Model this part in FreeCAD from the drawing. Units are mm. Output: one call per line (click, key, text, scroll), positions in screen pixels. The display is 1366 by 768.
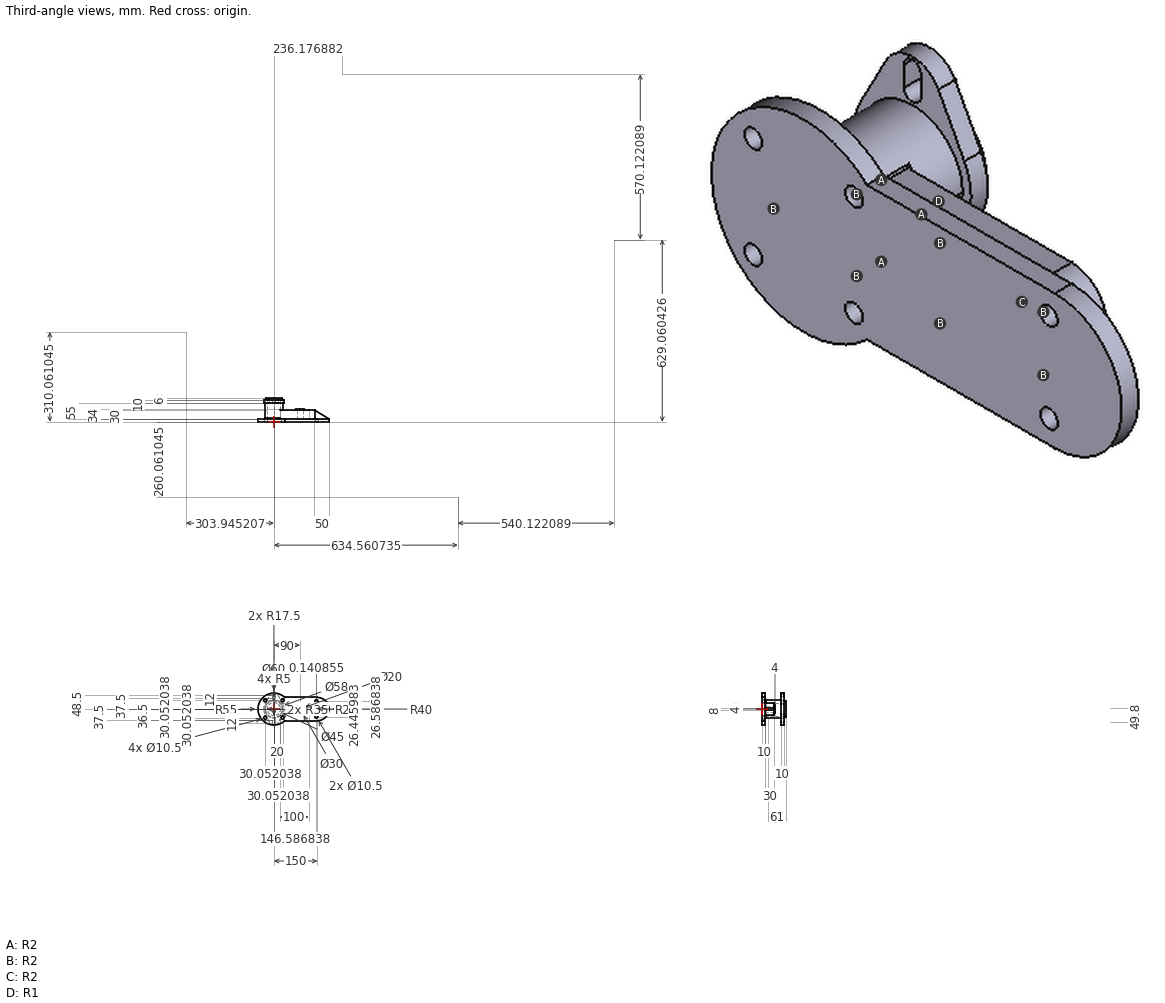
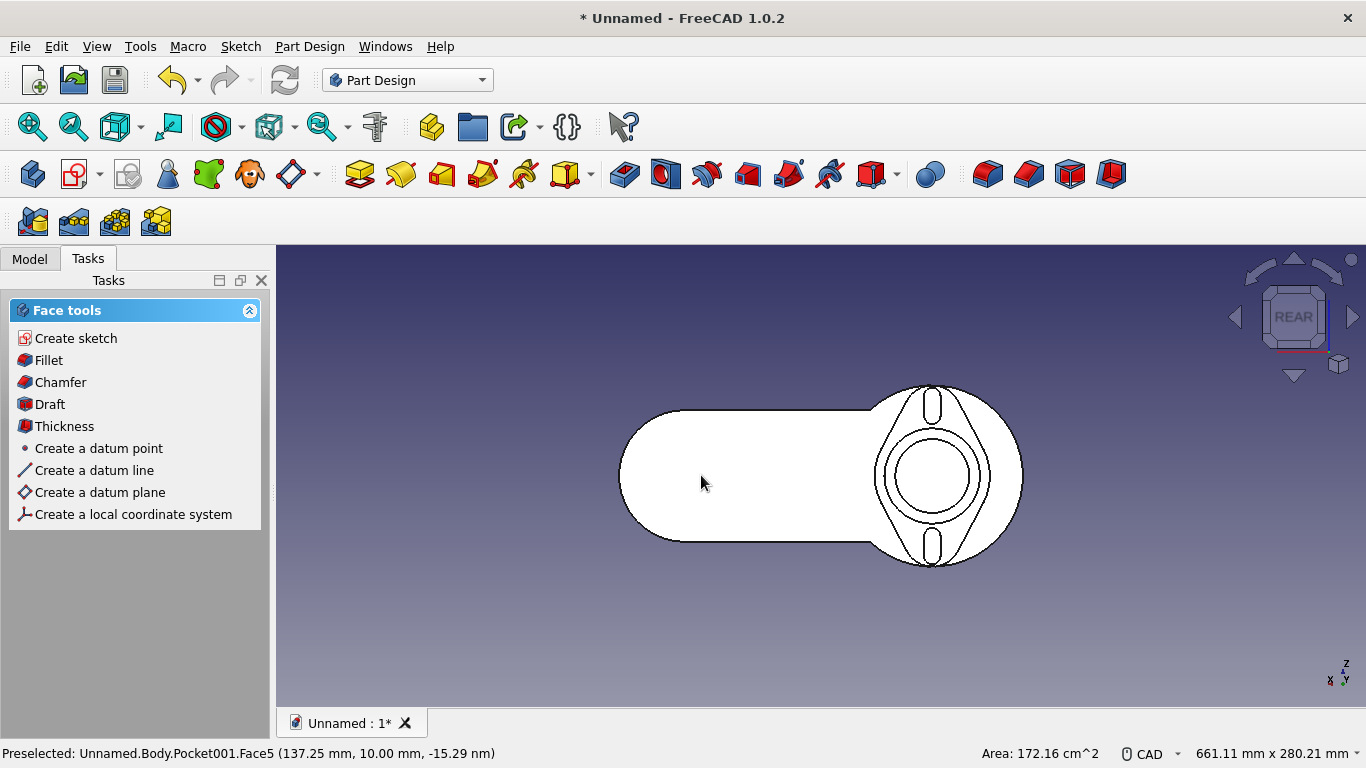
click(74, 174)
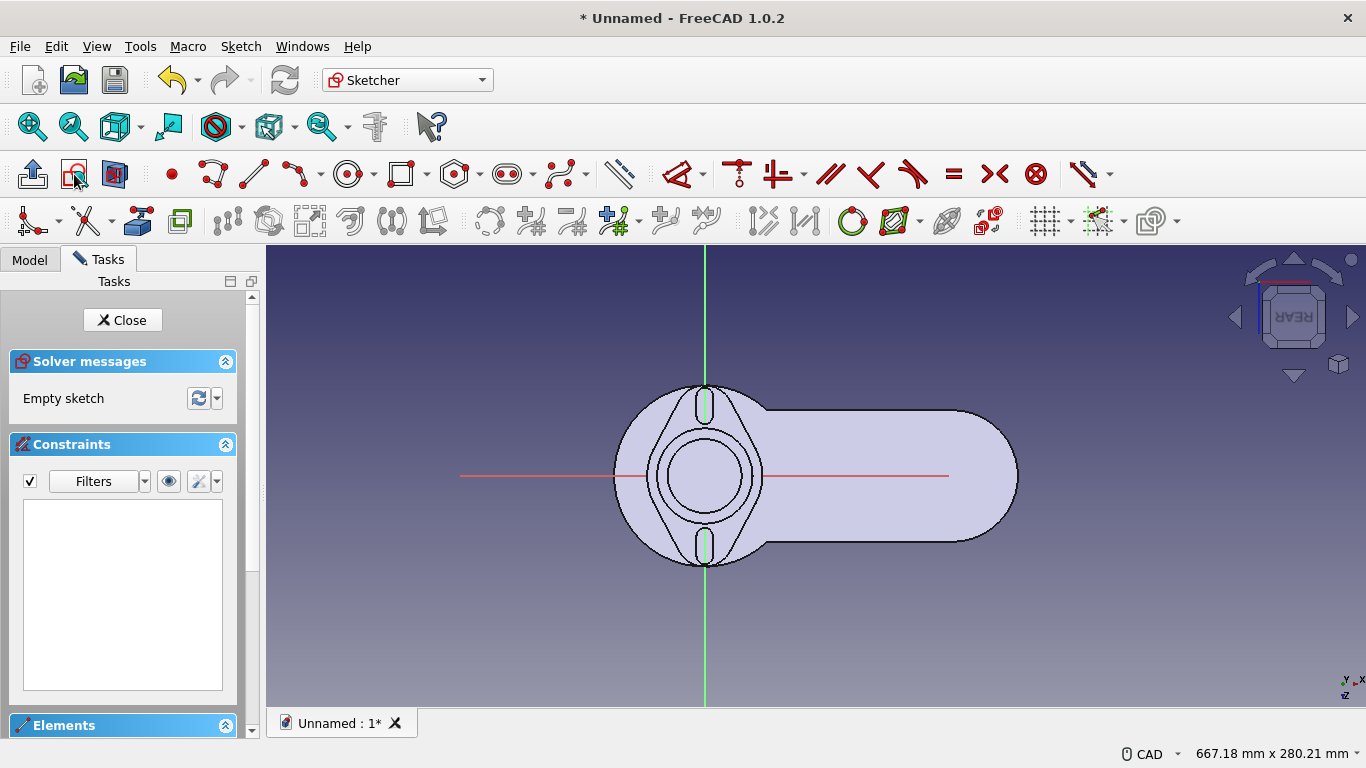
key(q)
key(s)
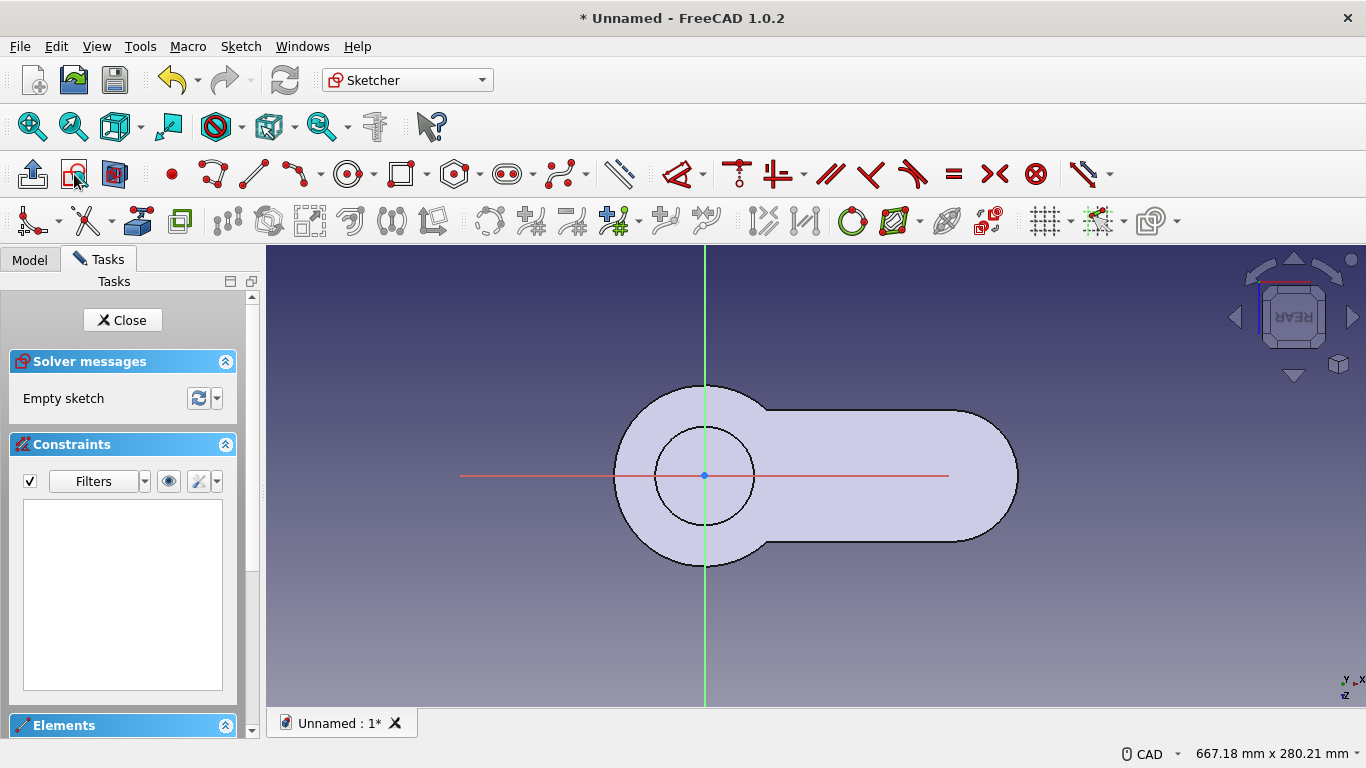
scroll(864, 476, up, 5)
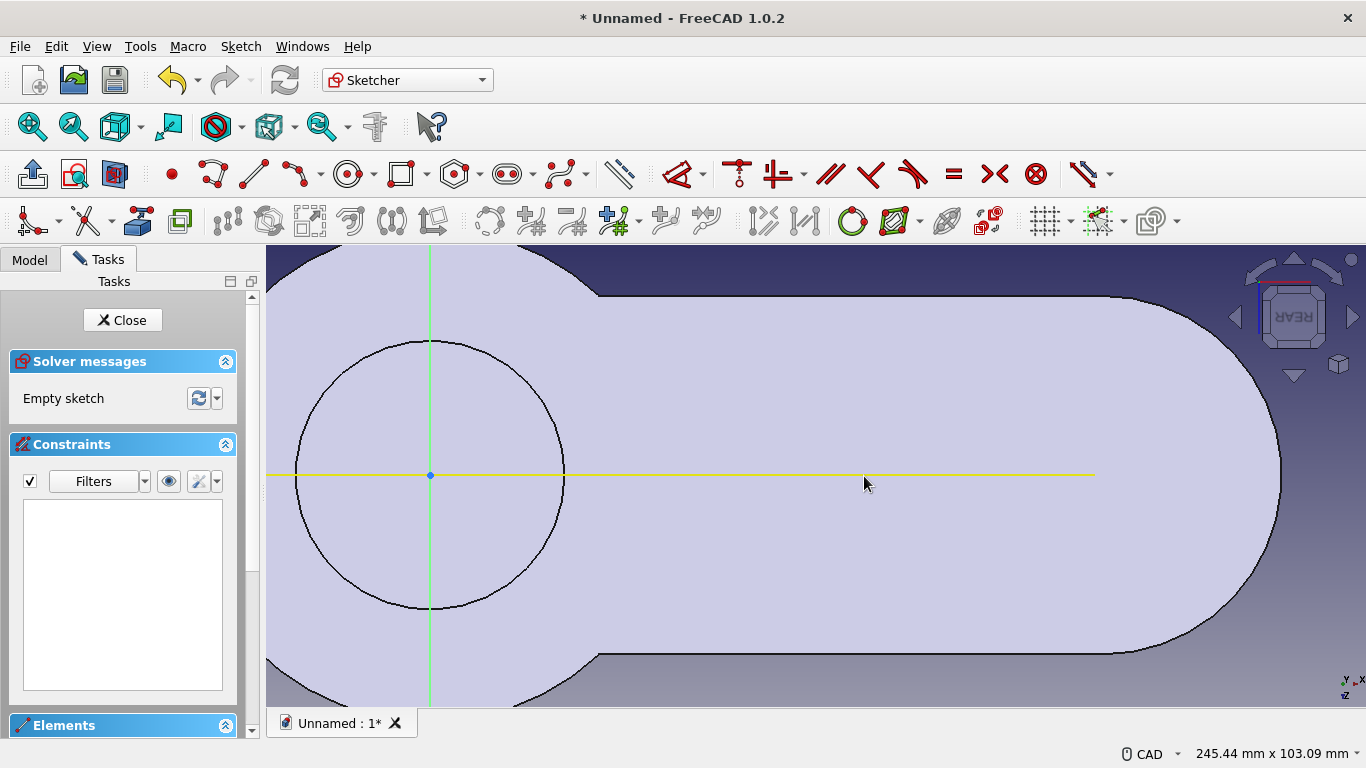
click(213, 174)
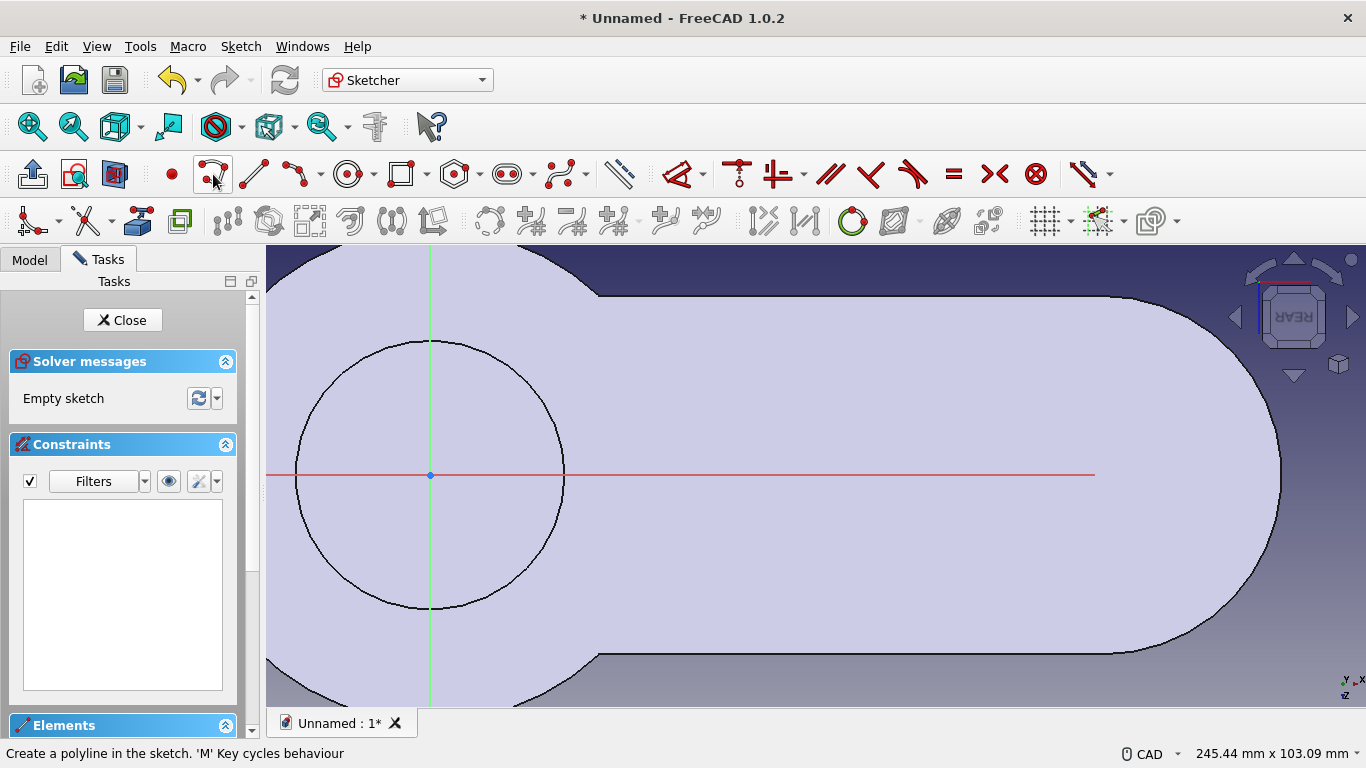
click(968, 381)
click(520, 381)
click(520, 569)
click(968, 569)
right_click(968, 569)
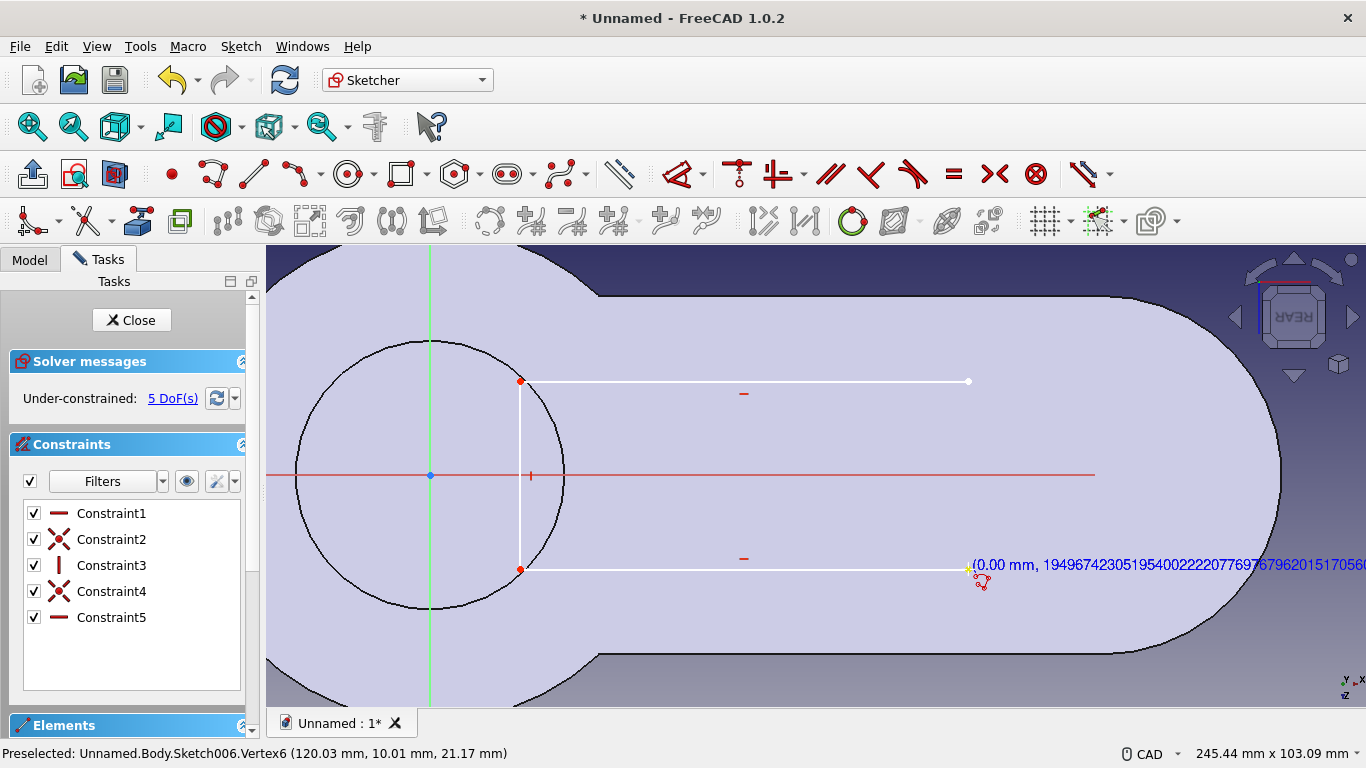
click(294, 174)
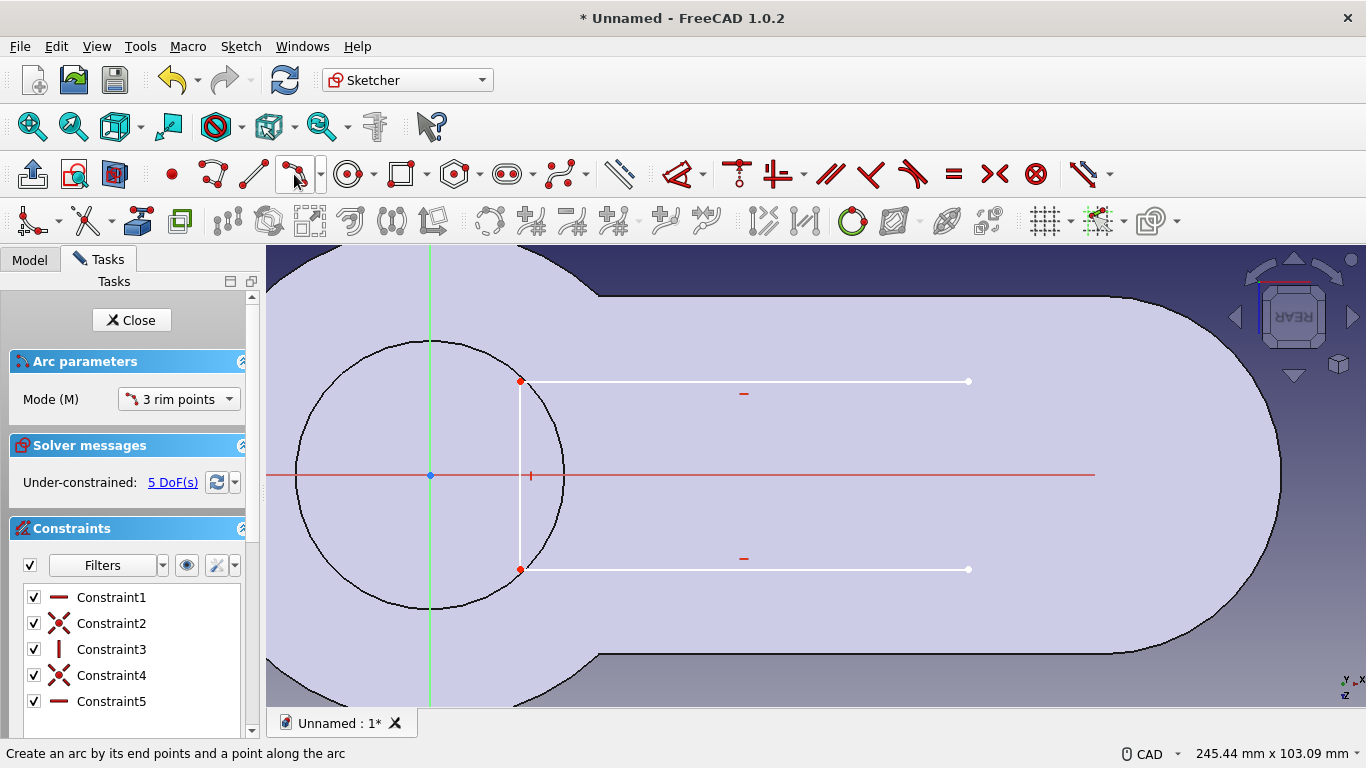
click(968, 570)
click(968, 382)
click(1057, 504)
key(Escape)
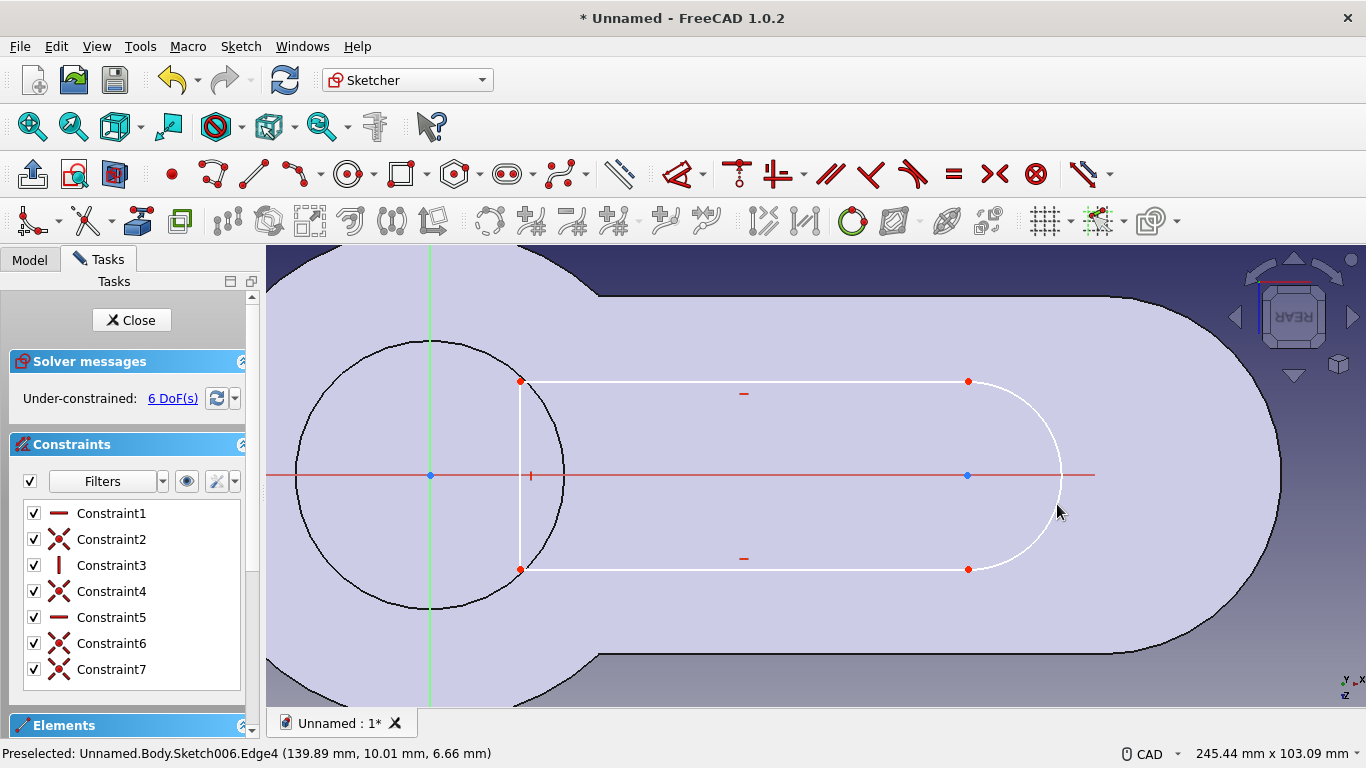
click(834, 382)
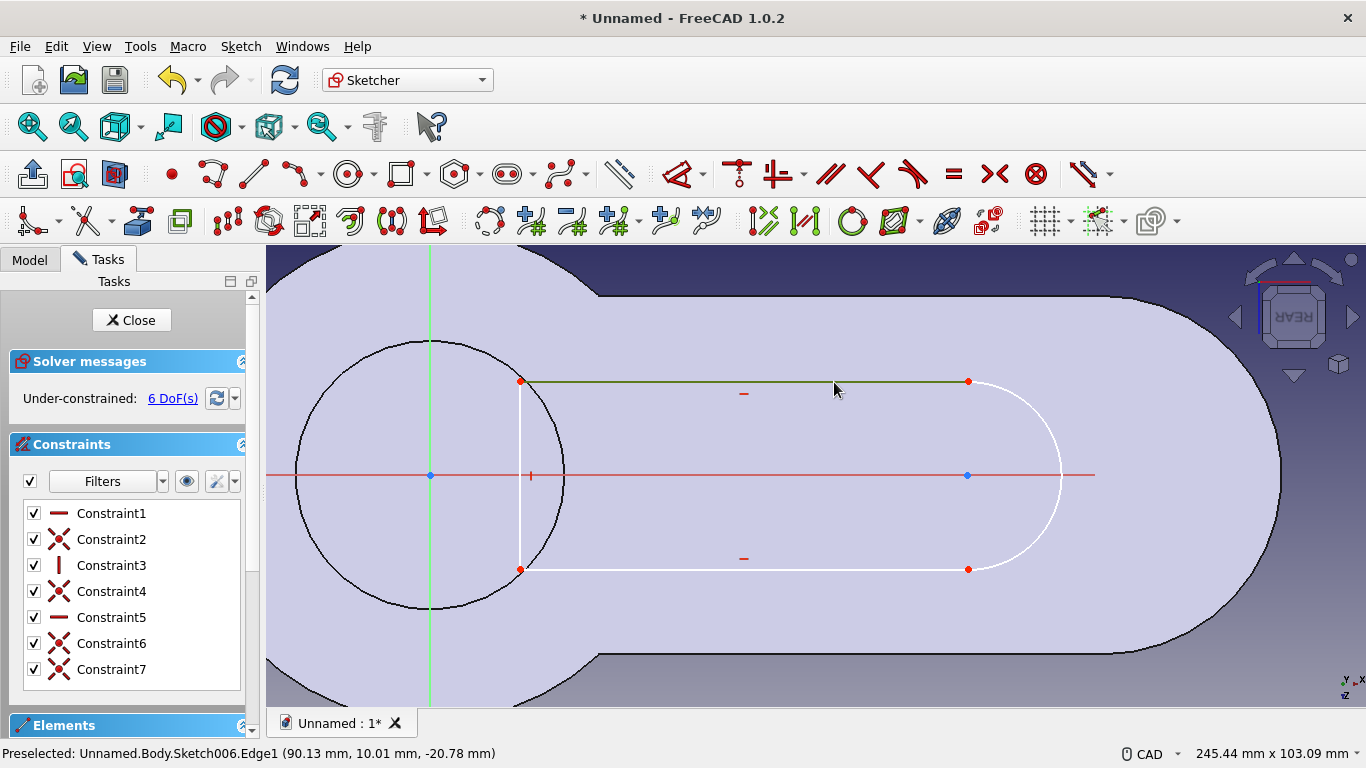
click(1044, 531)